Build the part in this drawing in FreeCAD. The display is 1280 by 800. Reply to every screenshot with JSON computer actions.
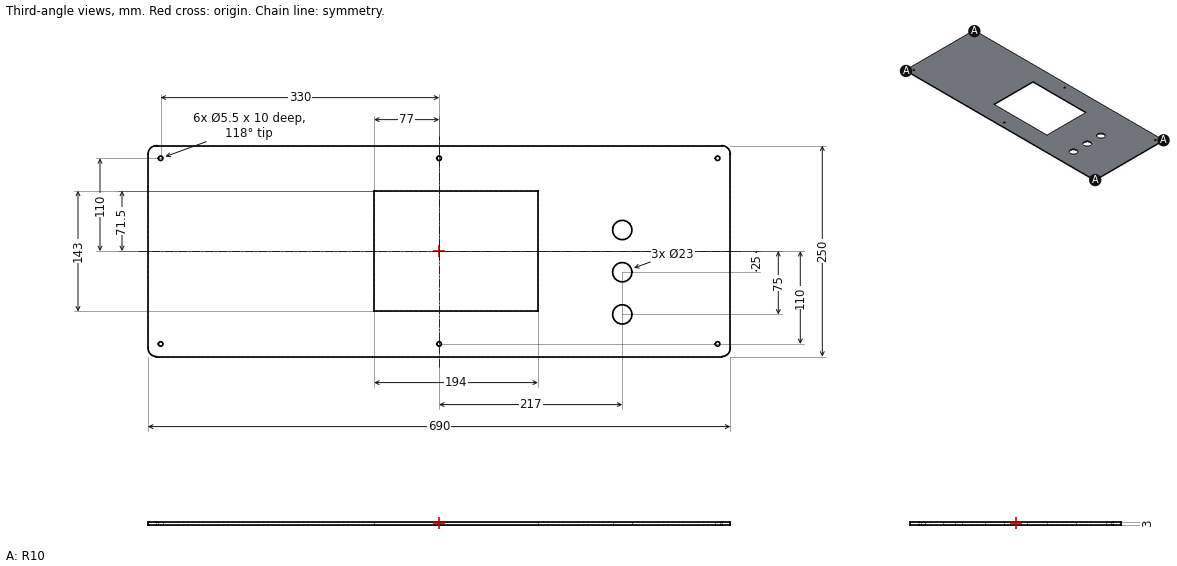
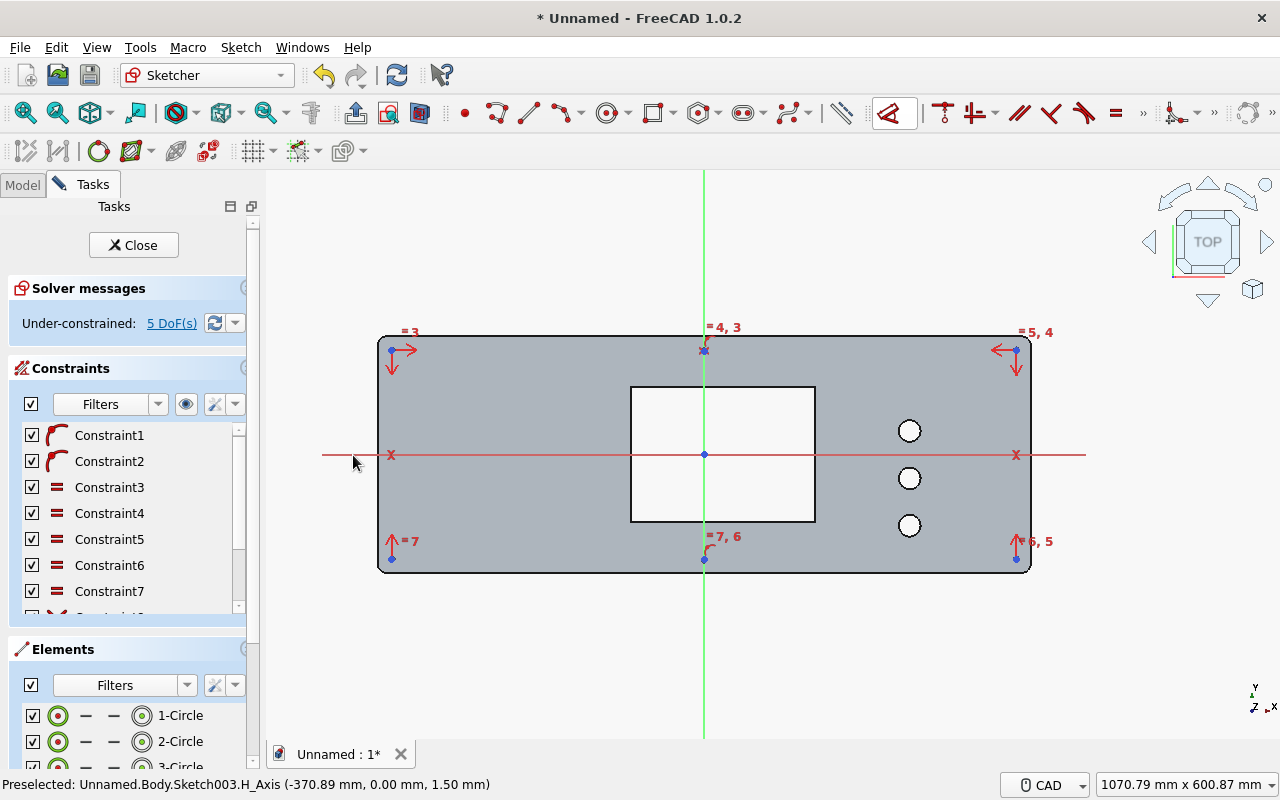
{"action": "scroll", "coordinate": [392, 348], "scroll_direction": "up", "scroll_amount": 11}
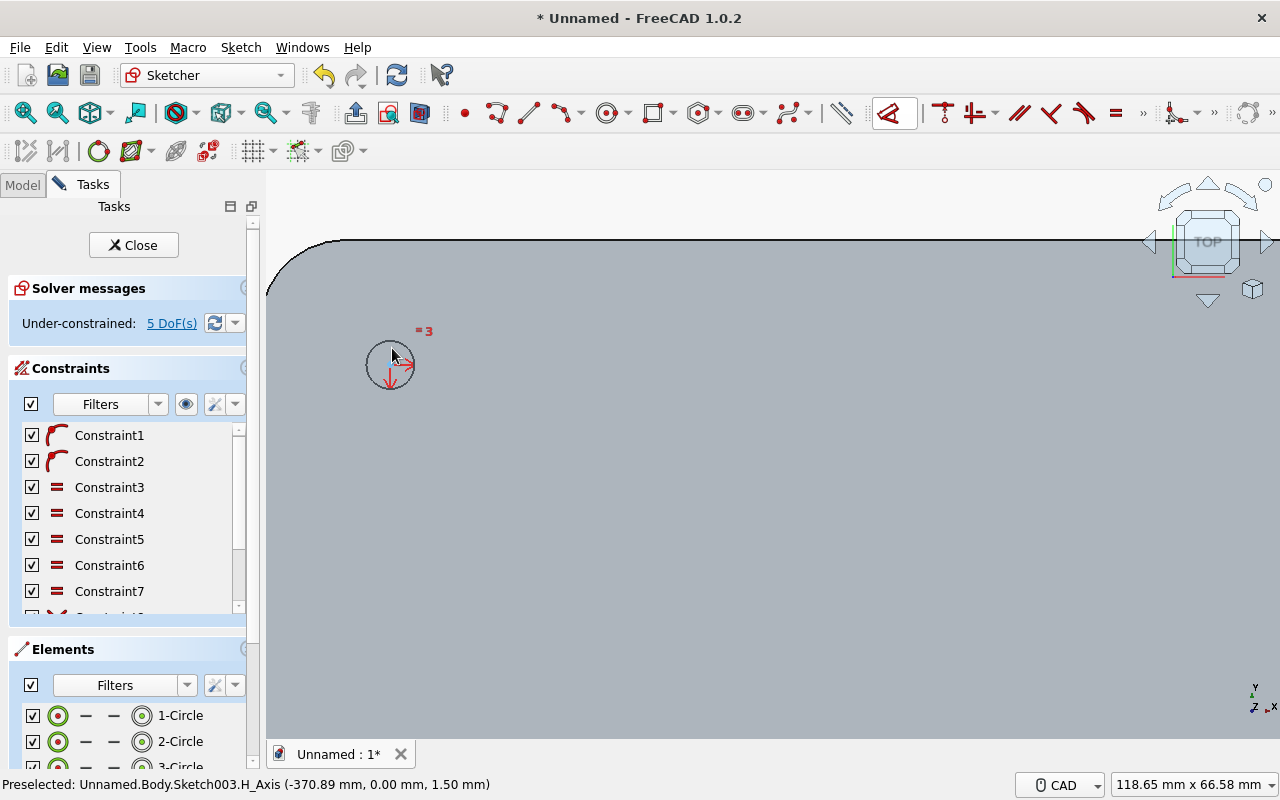
{"action": "left_click", "coordinate": [391, 341]}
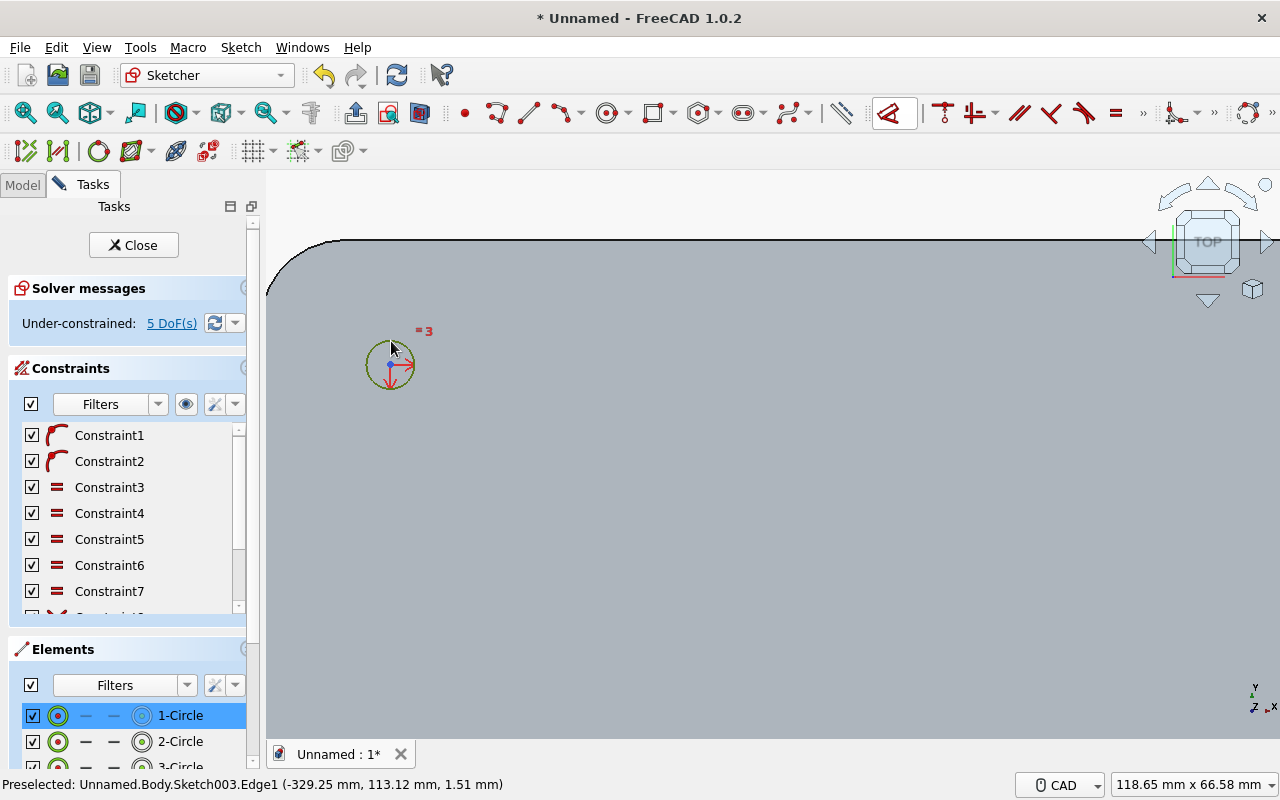
{"action": "key", "text": "k o"}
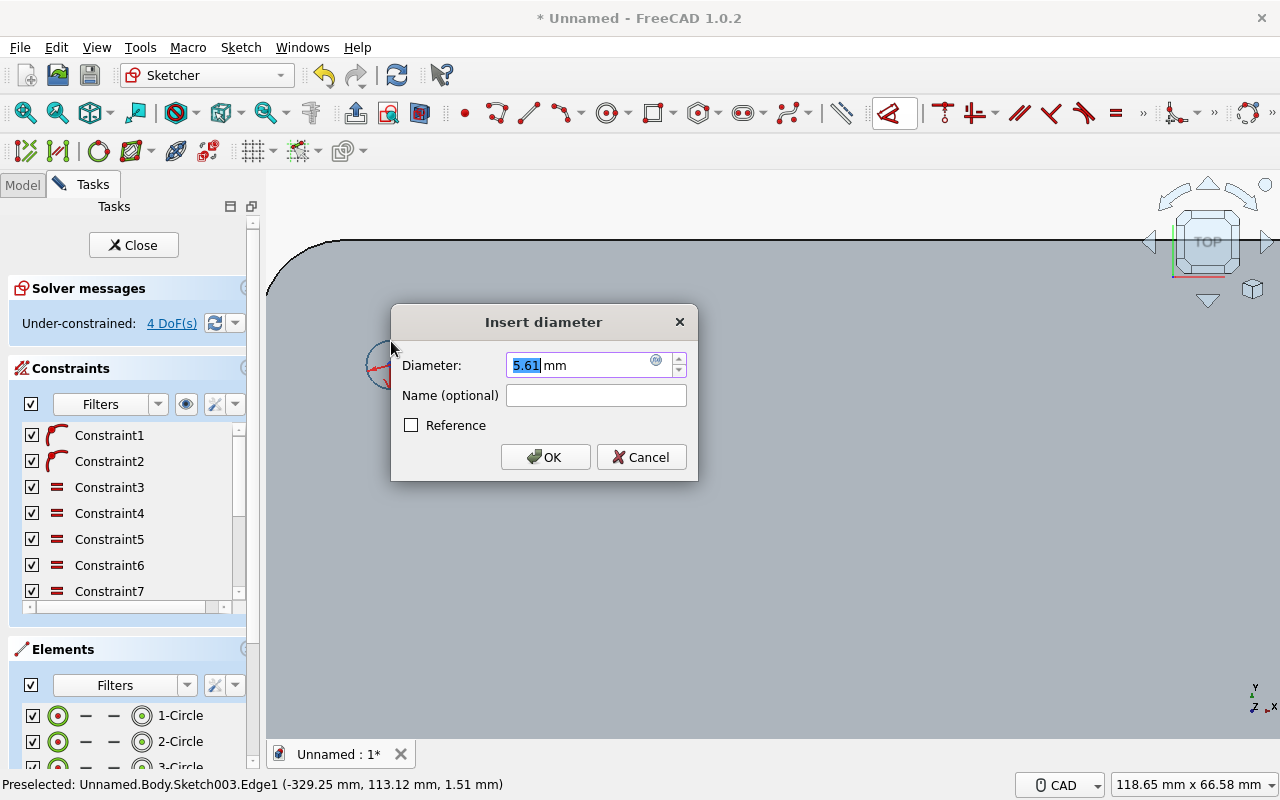
{"action": "type", "text": "5.5"}
{"action": "key", "text": "Return"}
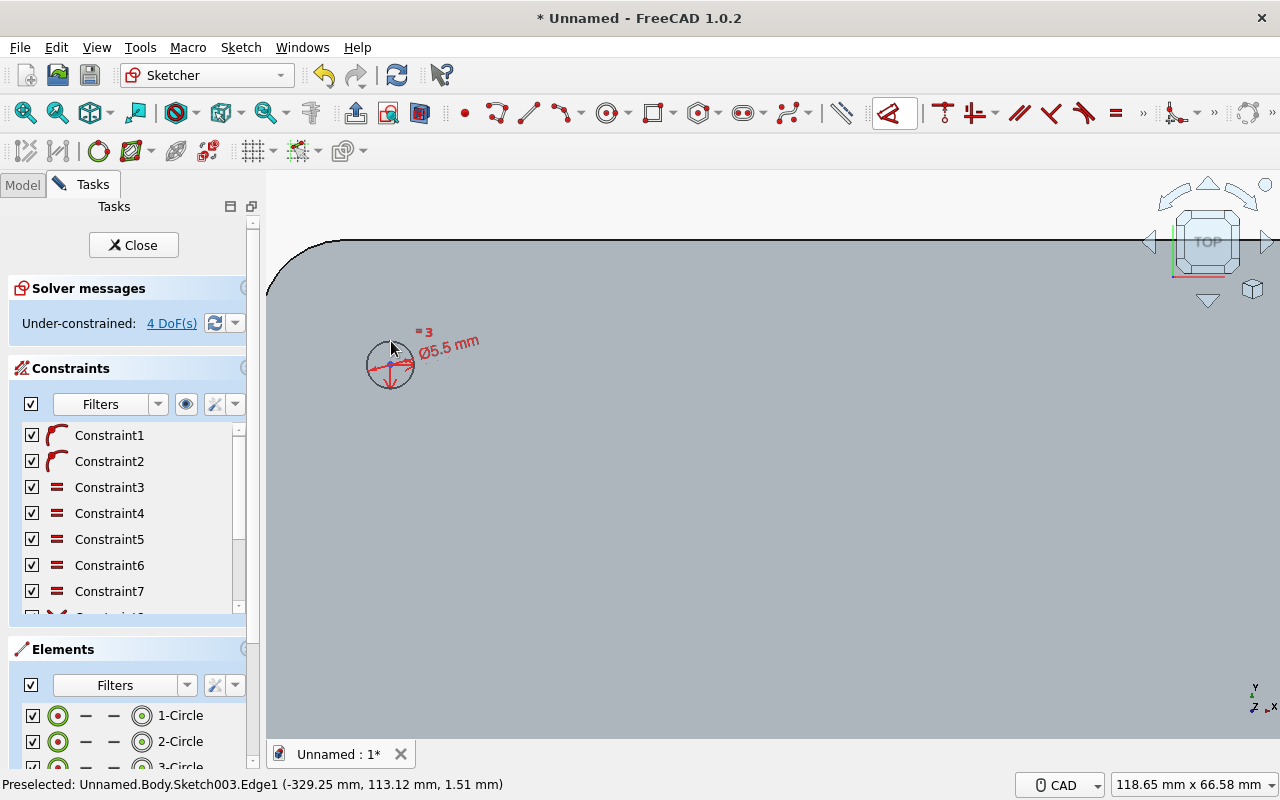
{"action": "scroll", "coordinate": [392, 348], "scroll_direction": "down", "scroll_amount": 11}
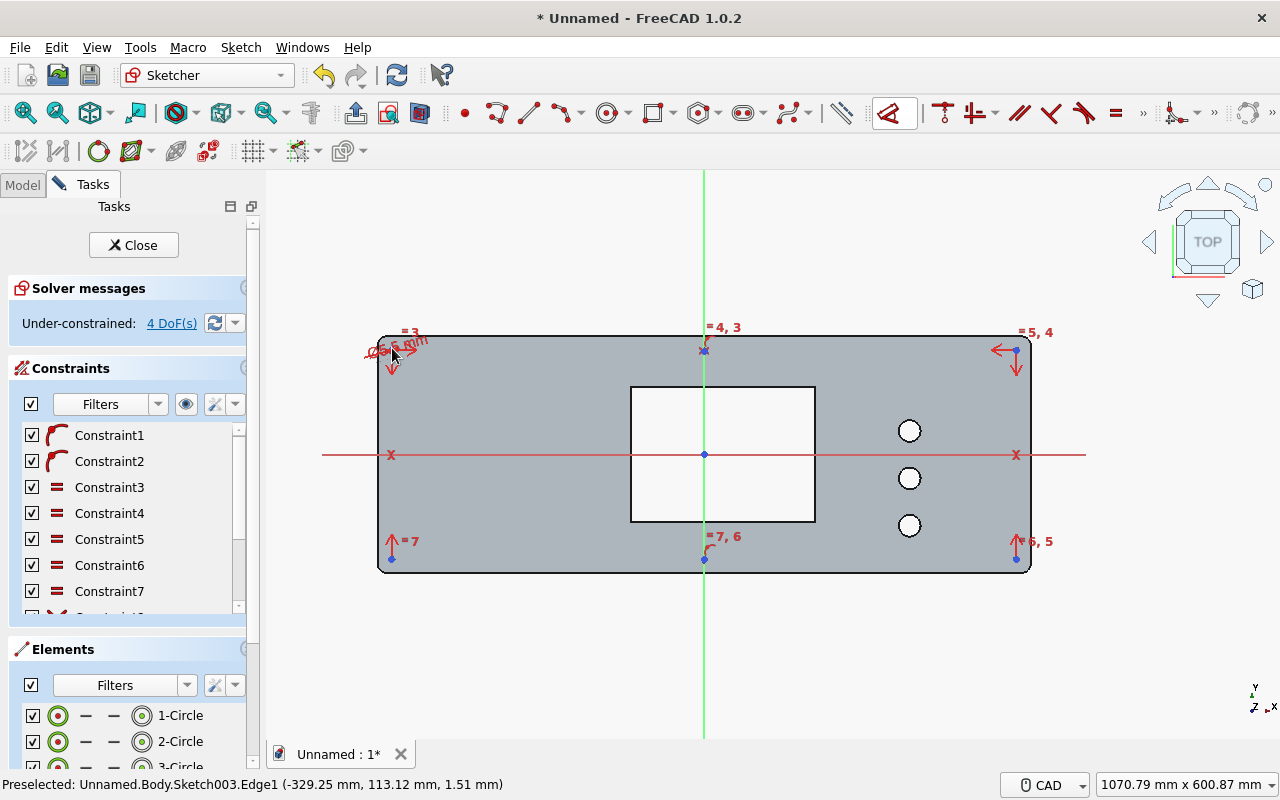
{"action": "left_click", "coordinate": [392, 350]}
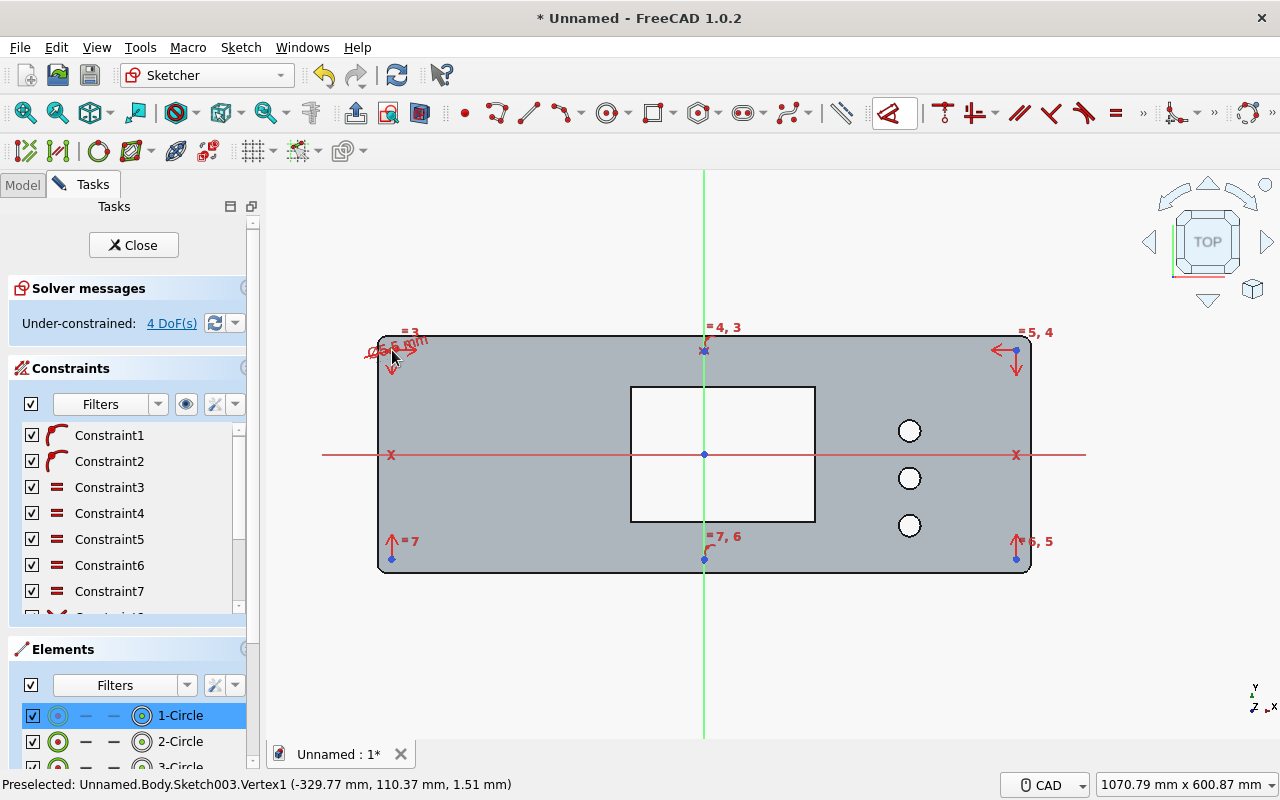
{"action": "key", "text": "l"}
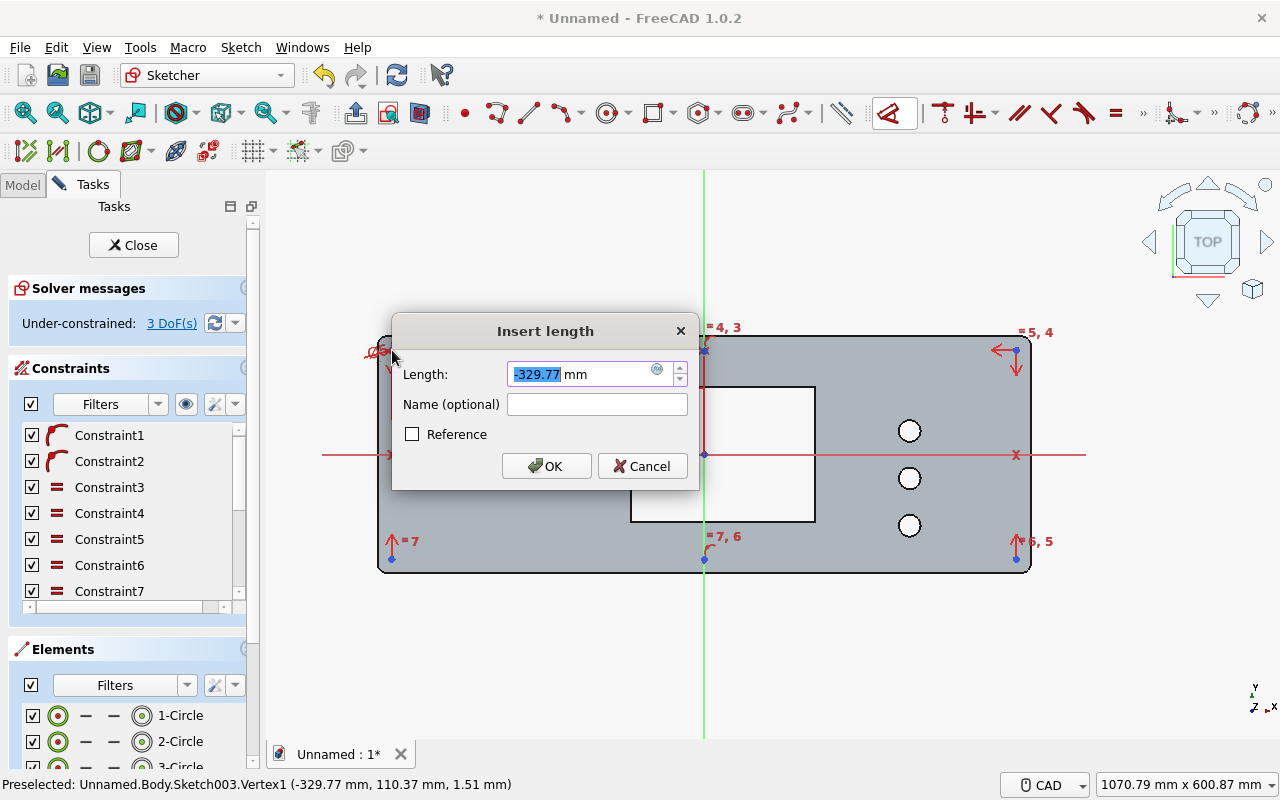
{"action": "type", "text": "-330"}
{"action": "key", "text": "Return"}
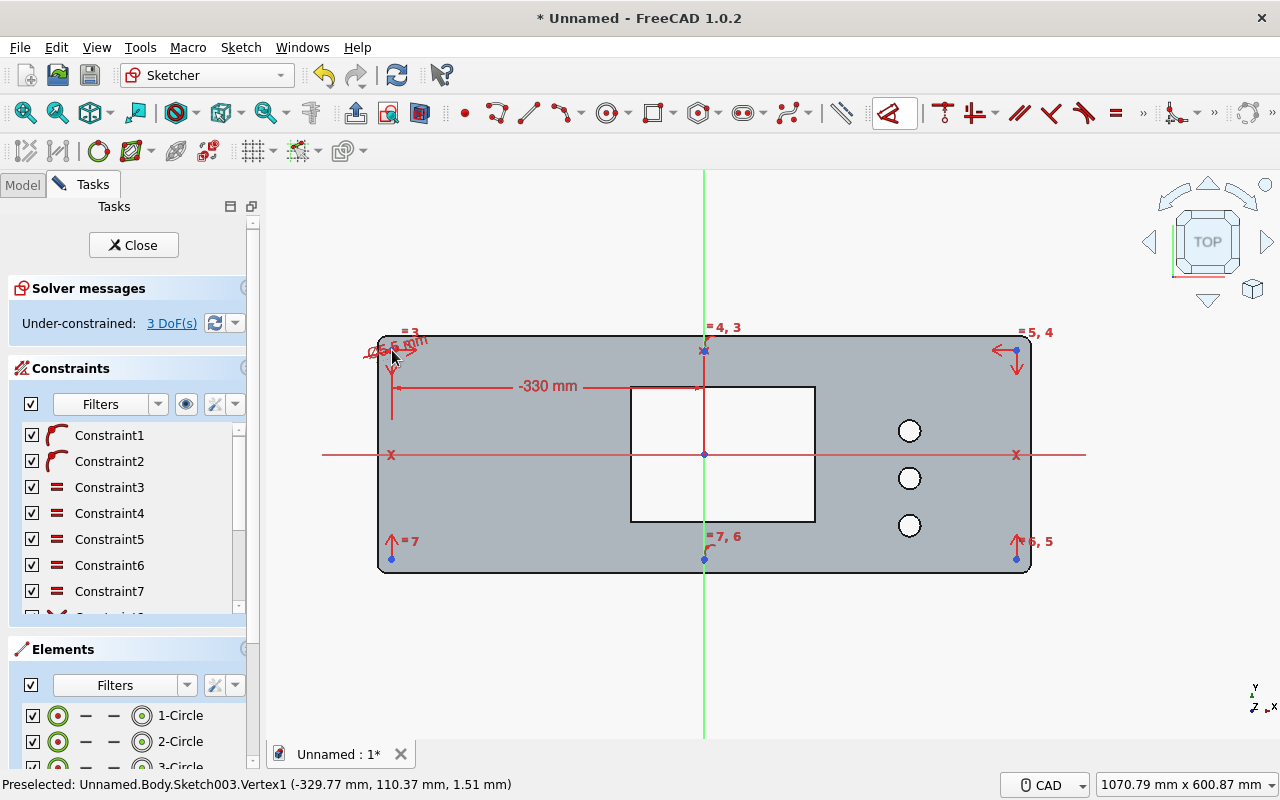
{"action": "left_click", "coordinate": [392, 350]}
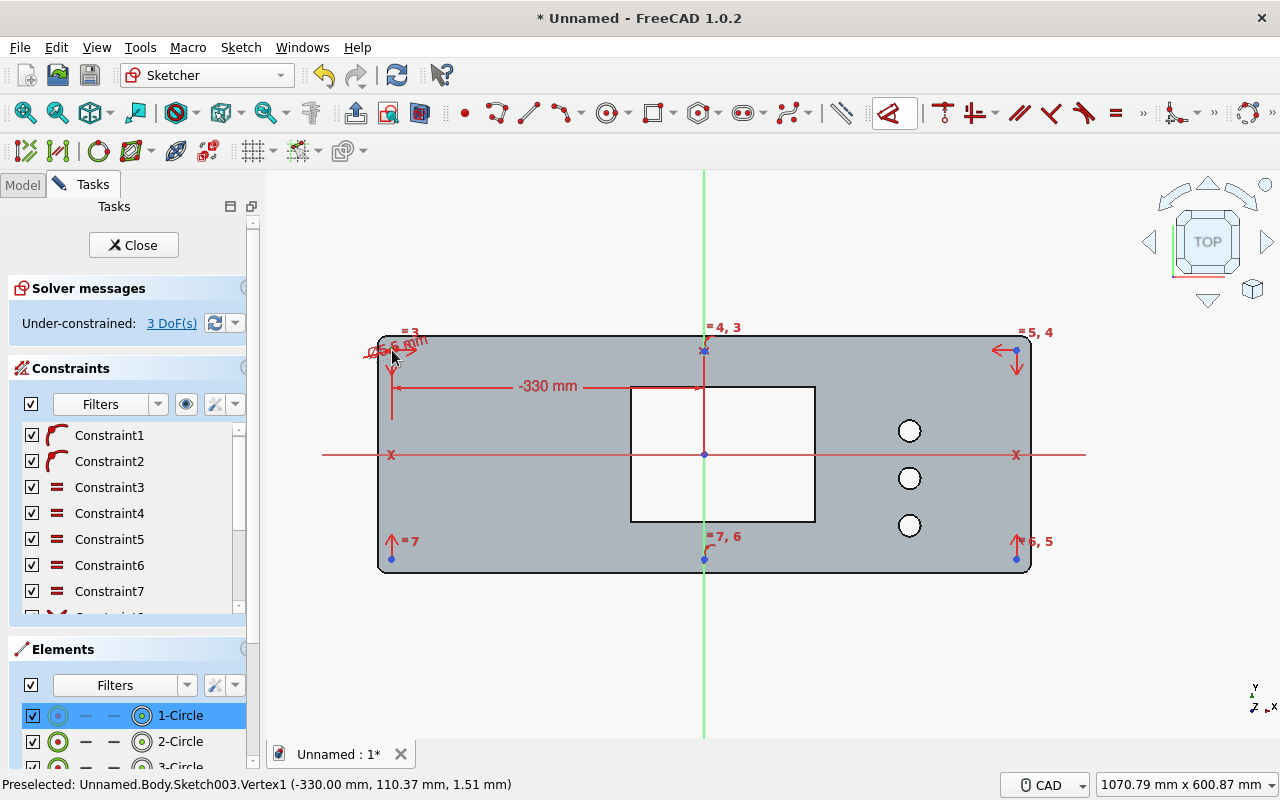
{"action": "key", "text": "i"}